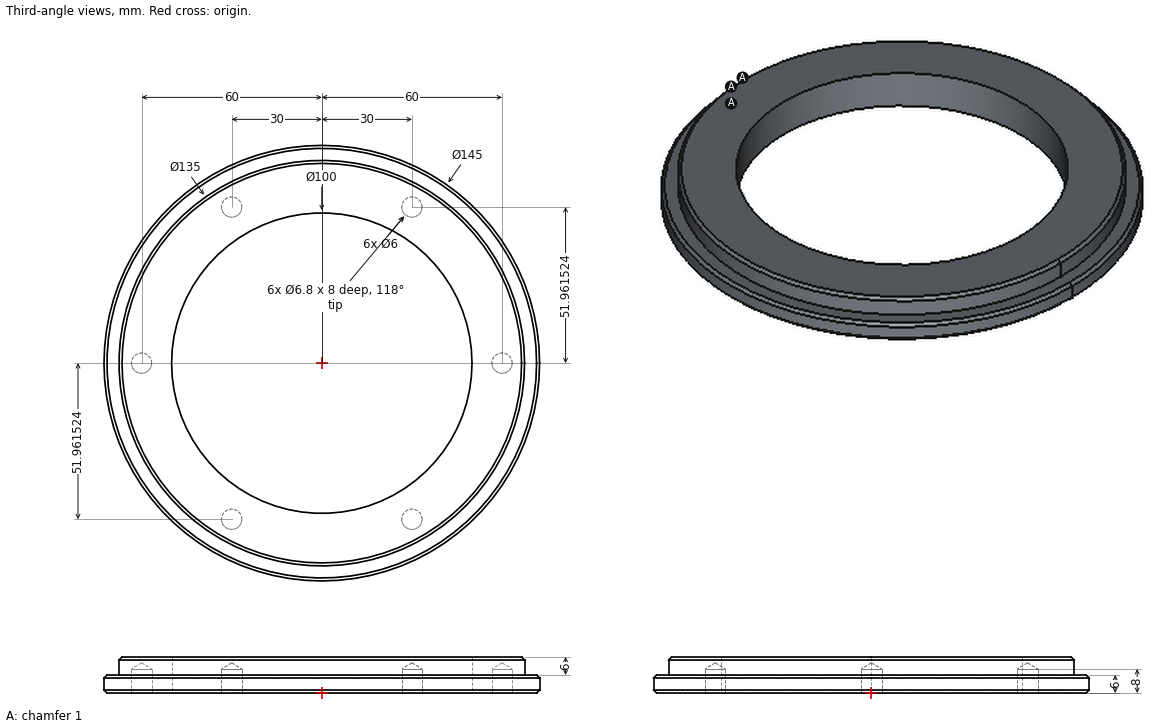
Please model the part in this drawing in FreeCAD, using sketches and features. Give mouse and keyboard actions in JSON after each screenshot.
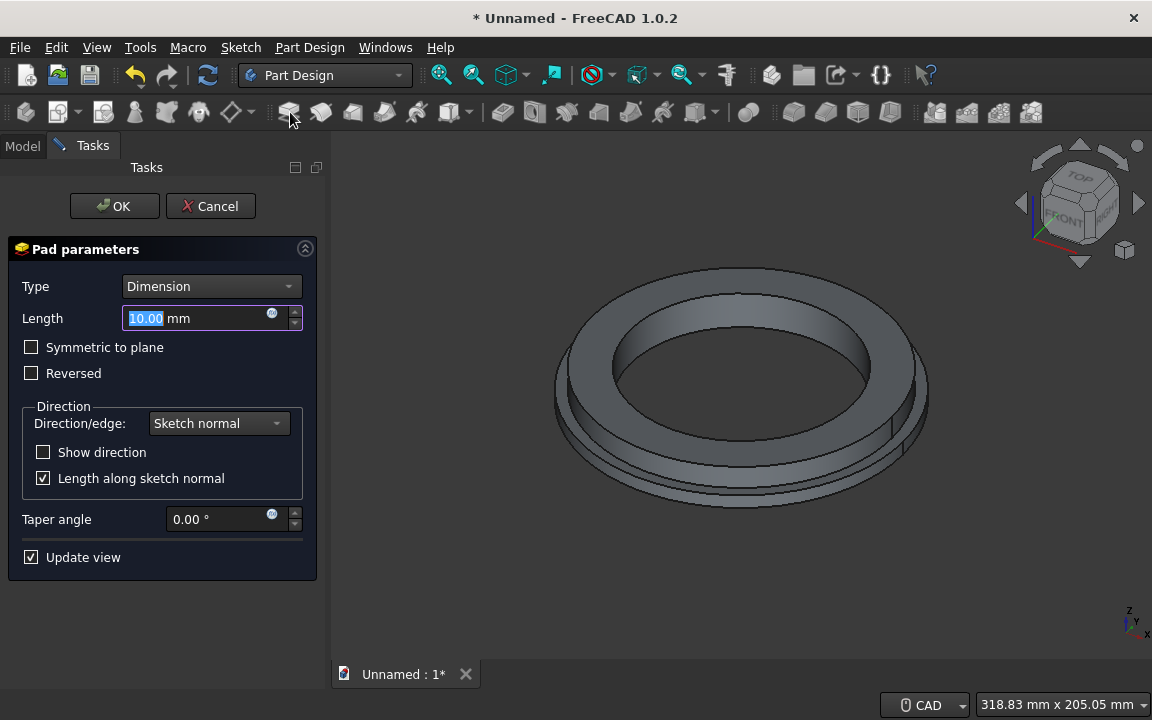
{"action": "type", "text": "6"}
{"action": "key", "text": "Tab"}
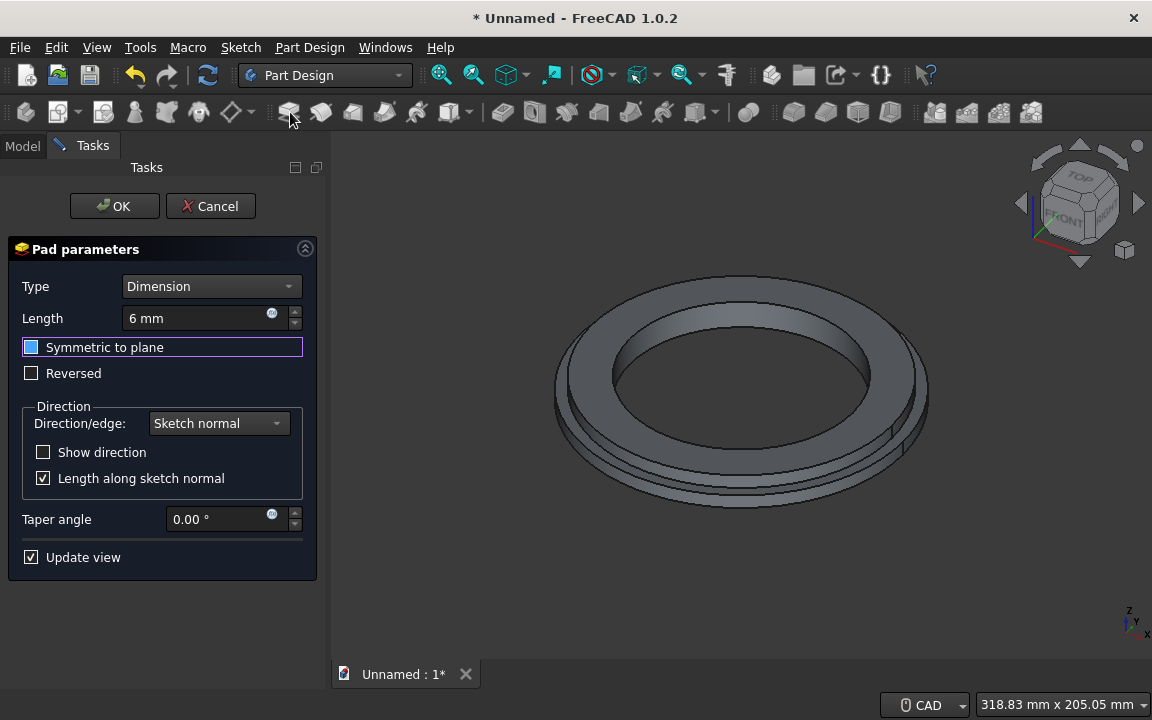
{"action": "left_click", "coordinate": [115, 206]}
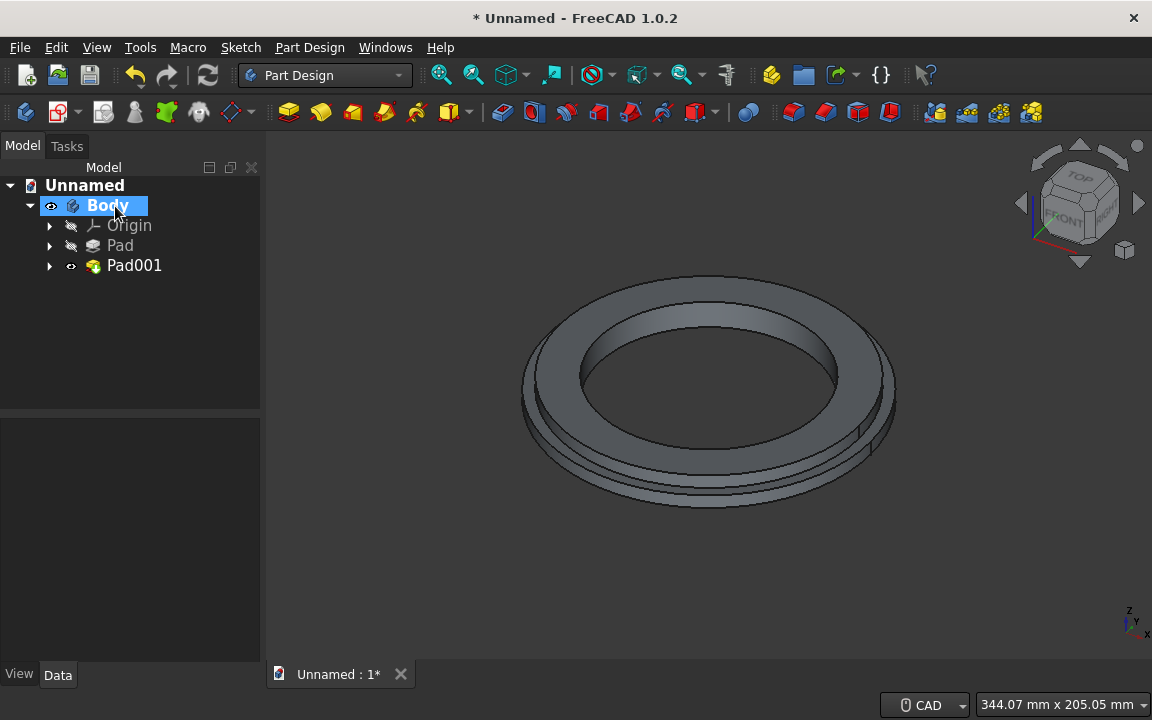
{"action": "left_click", "coordinate": [536, 385]}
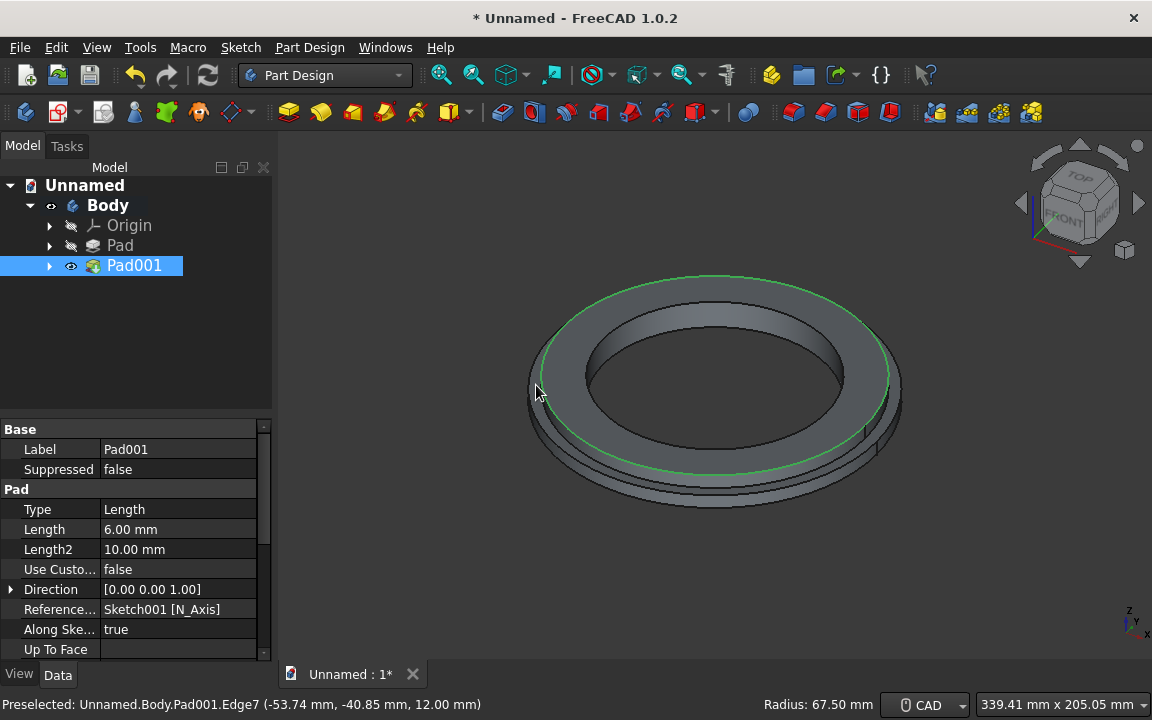
{"action": "left_click", "coordinate": [529, 399], "text": "ctrl"}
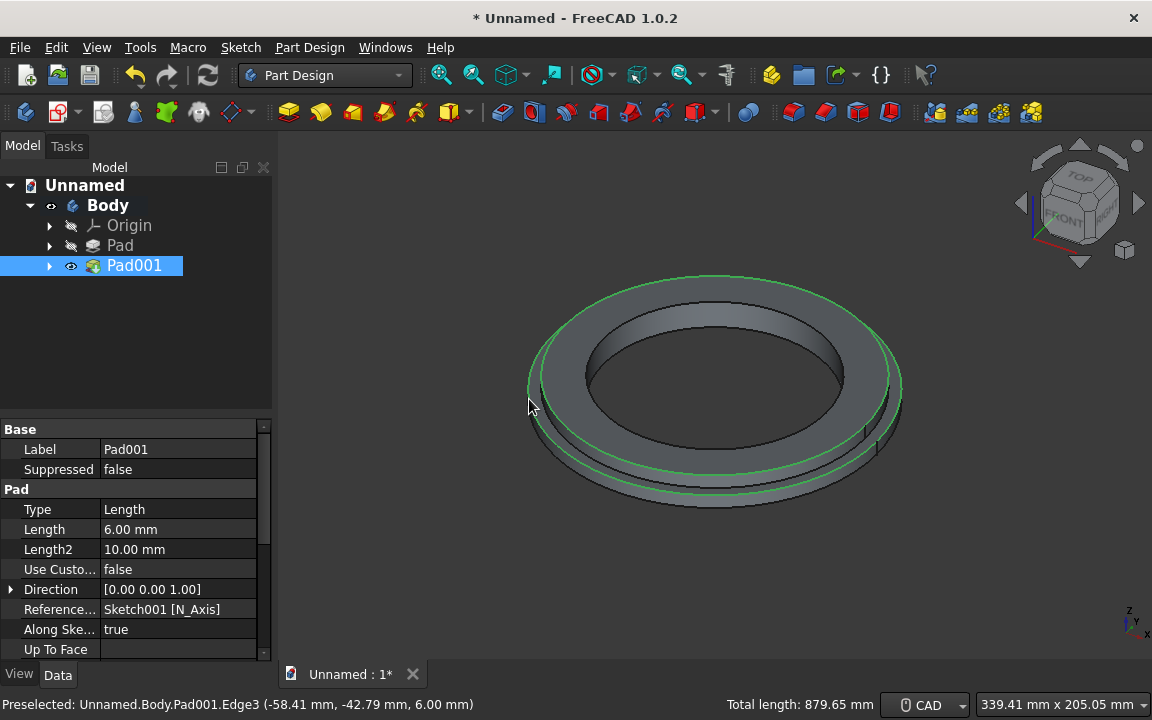
{"action": "key", "text": "0"}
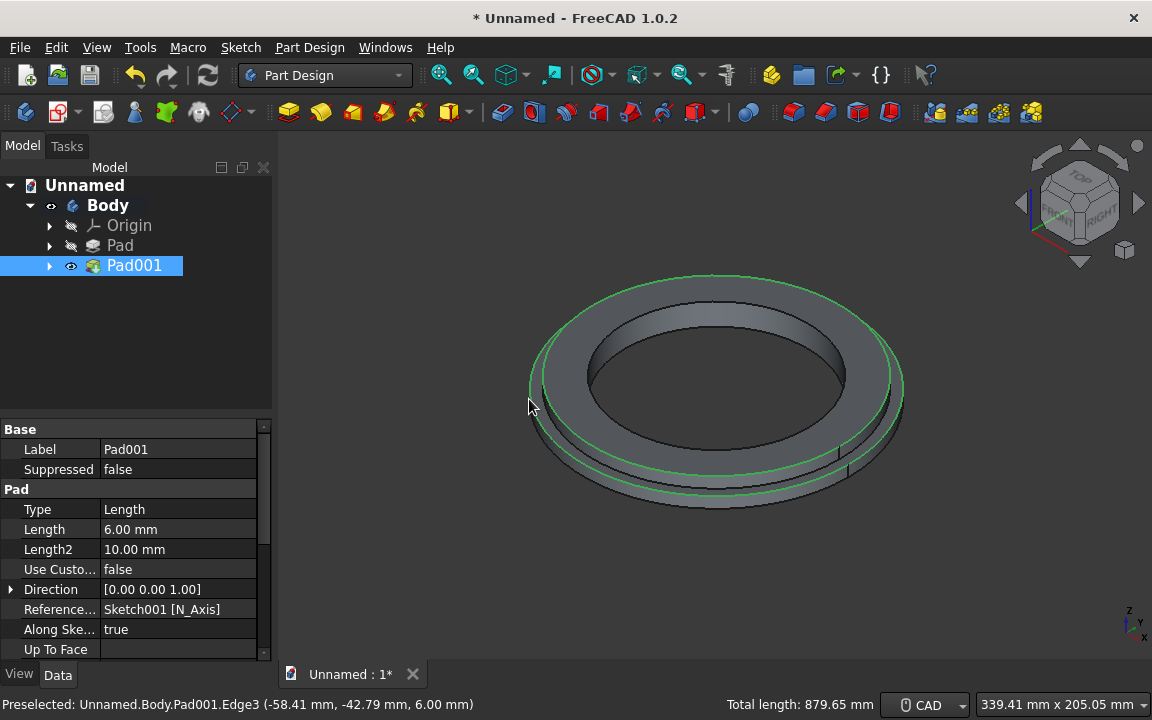
{"action": "left_click", "coordinate": [632, 496], "text": "ctrl"}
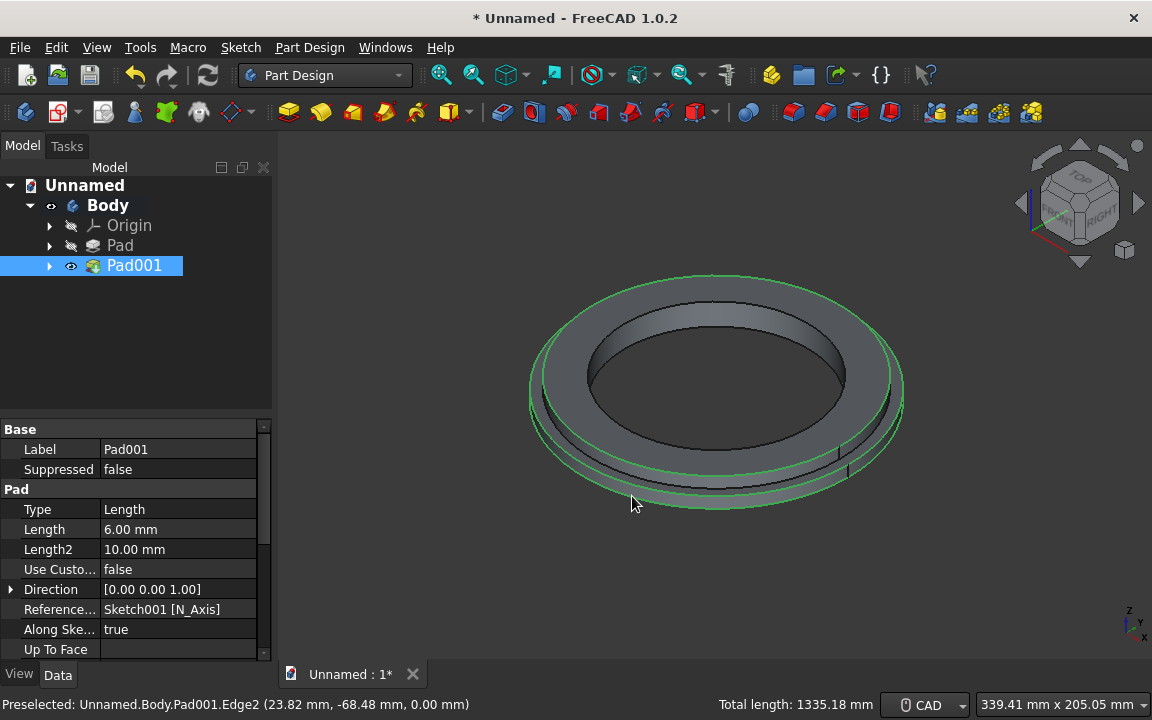
{"action": "left_click", "coordinate": [826, 112]}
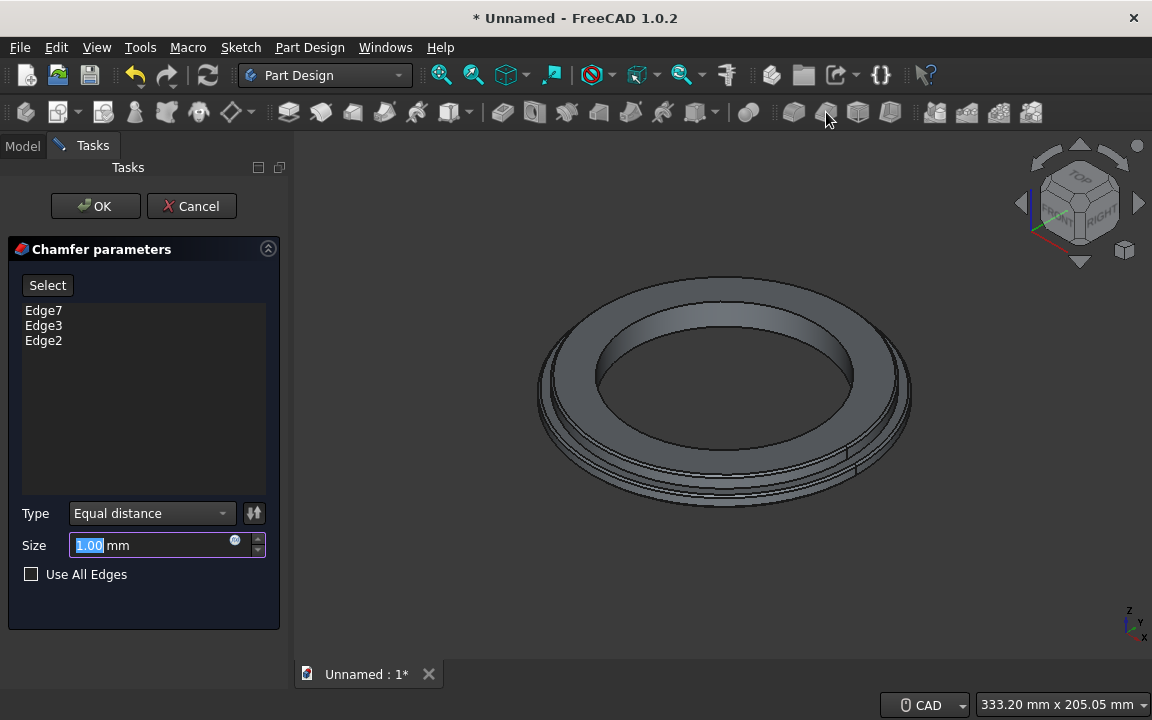
{"action": "type", "text": "1"}
{"action": "key", "text": "Tab"}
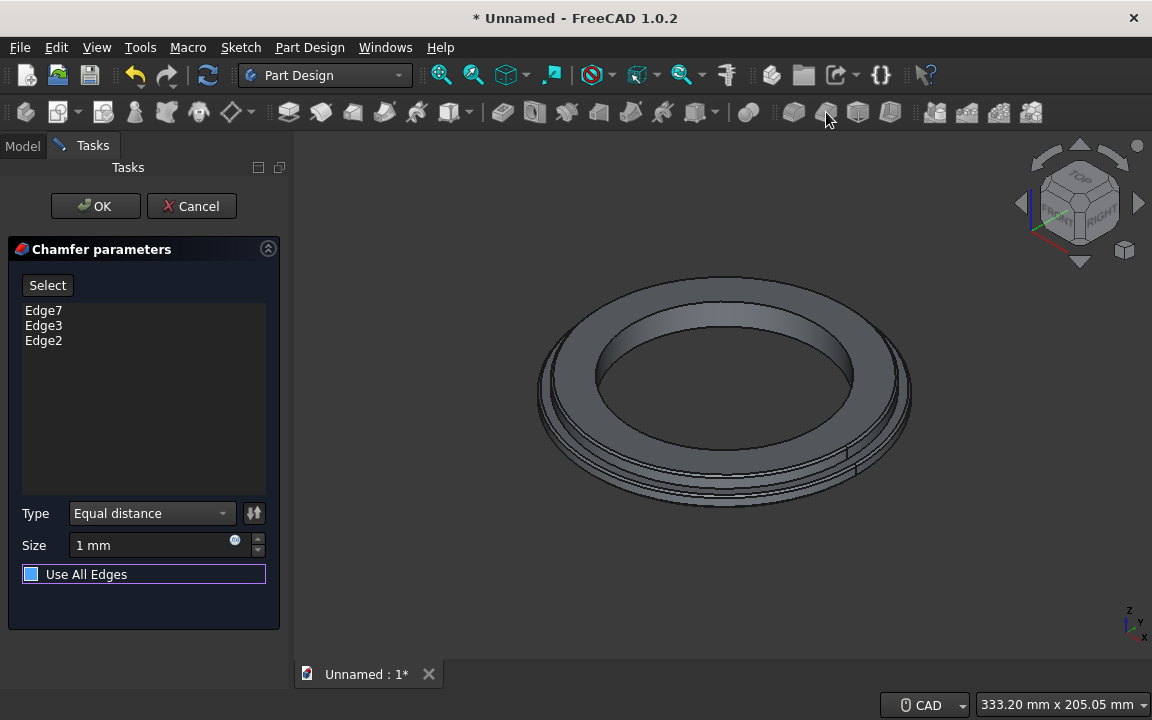
{"action": "left_click", "coordinate": [96, 206]}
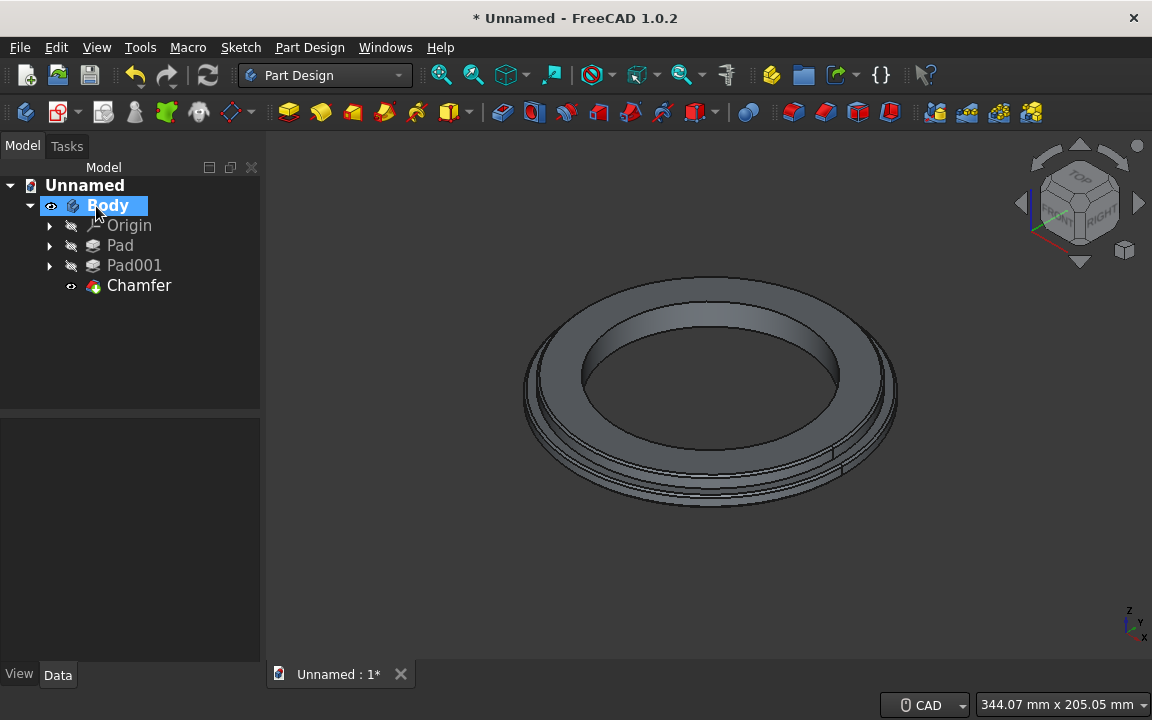
{"action": "key", "text": "5"}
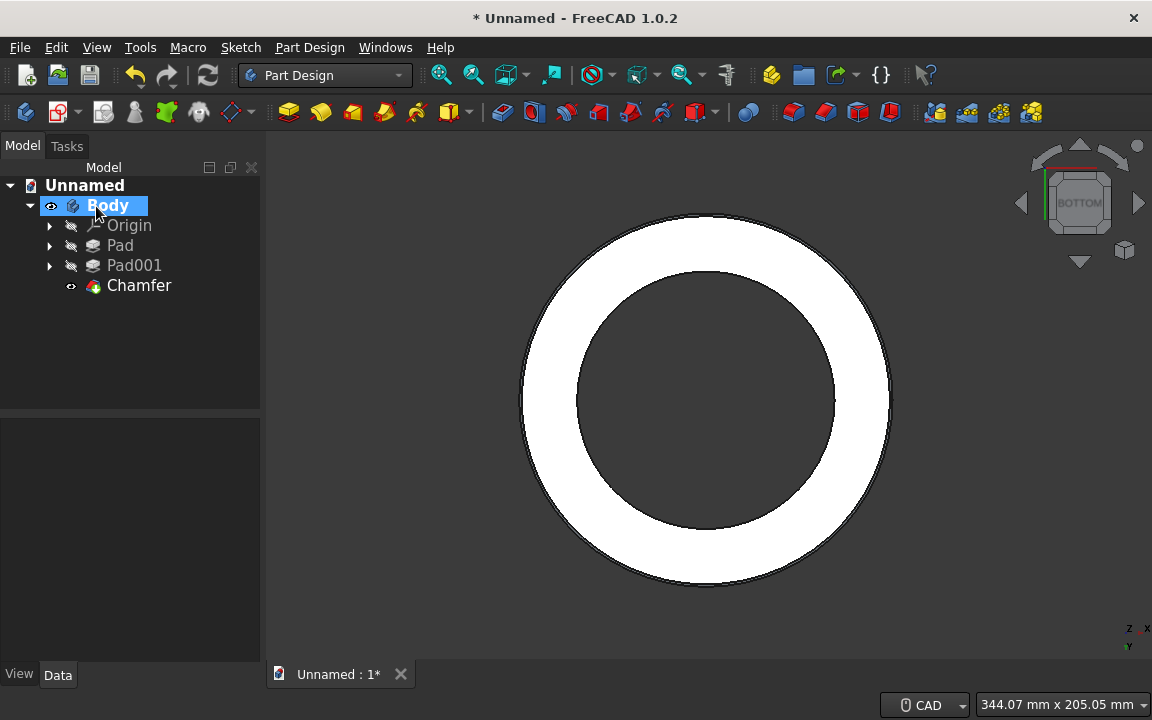
{"action": "left_click", "coordinate": [864, 399]}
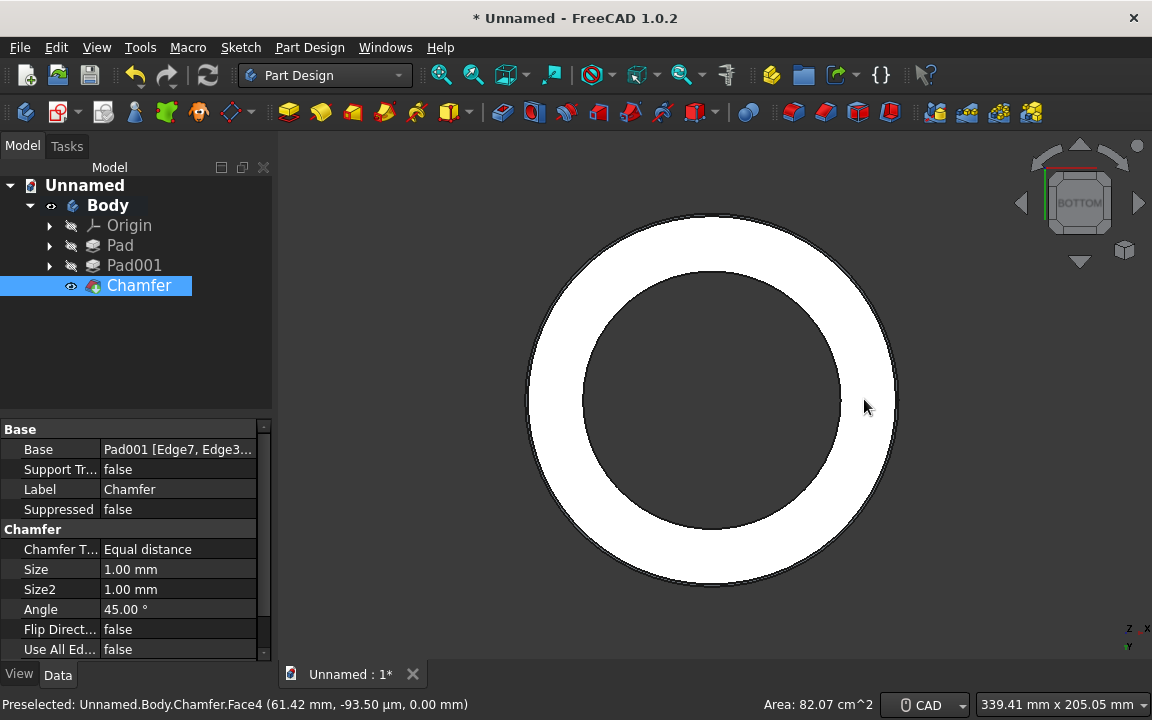
{"action": "left_click", "coordinate": [58, 112]}